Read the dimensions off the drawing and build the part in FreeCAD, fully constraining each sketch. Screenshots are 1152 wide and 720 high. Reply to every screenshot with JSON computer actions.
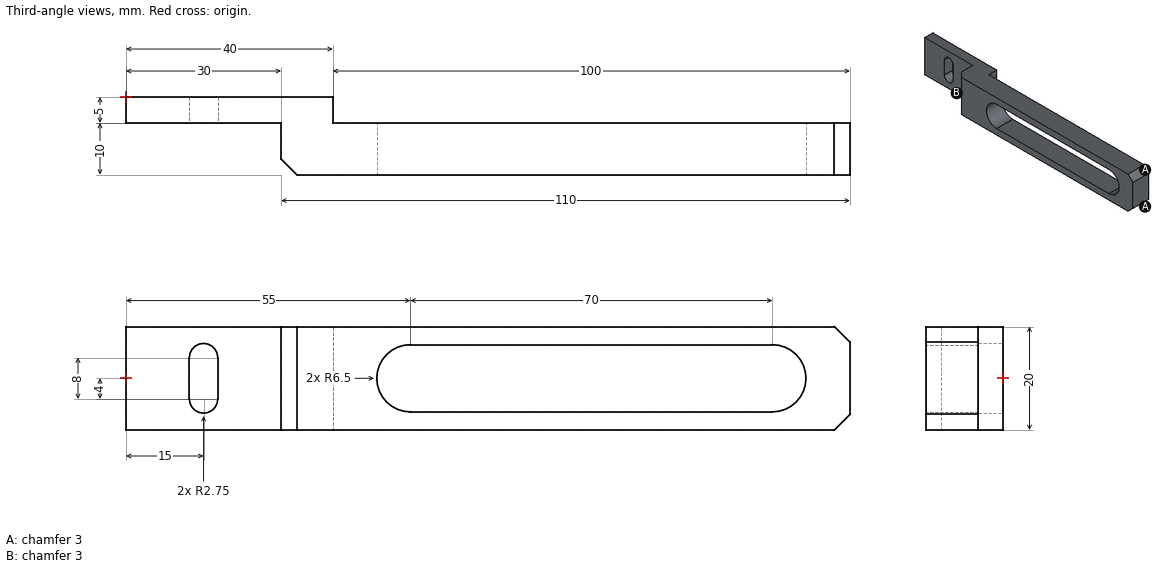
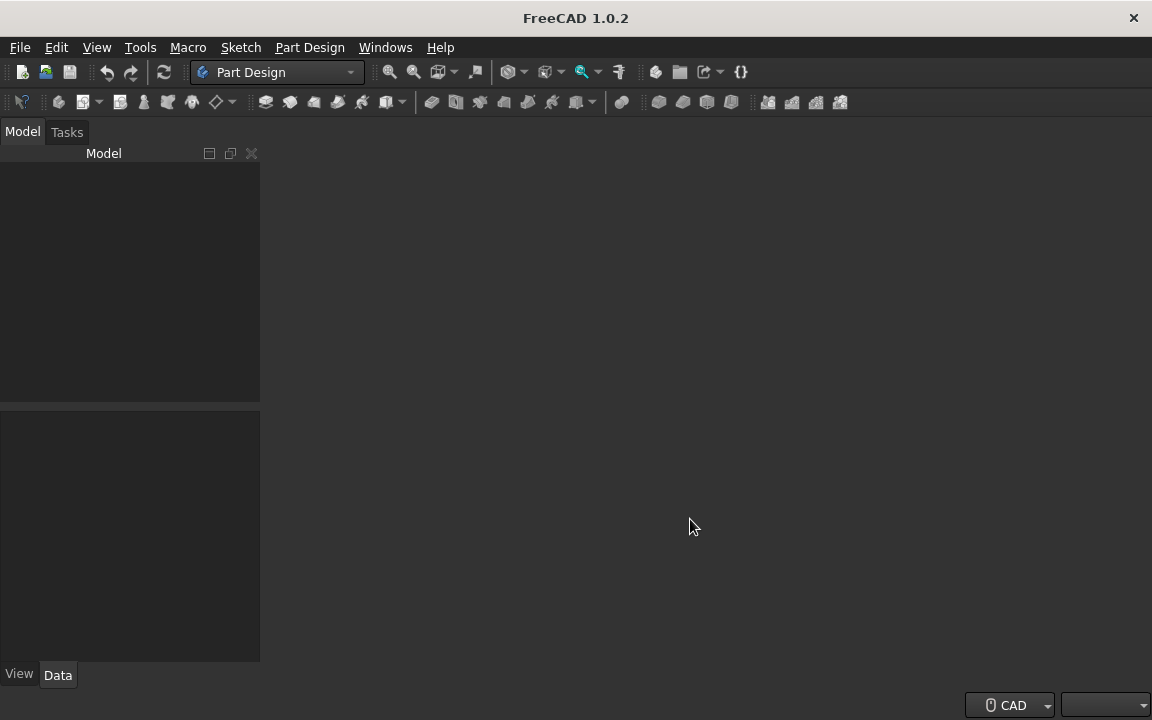
{"action": "left_click", "coordinate": [22, 72]}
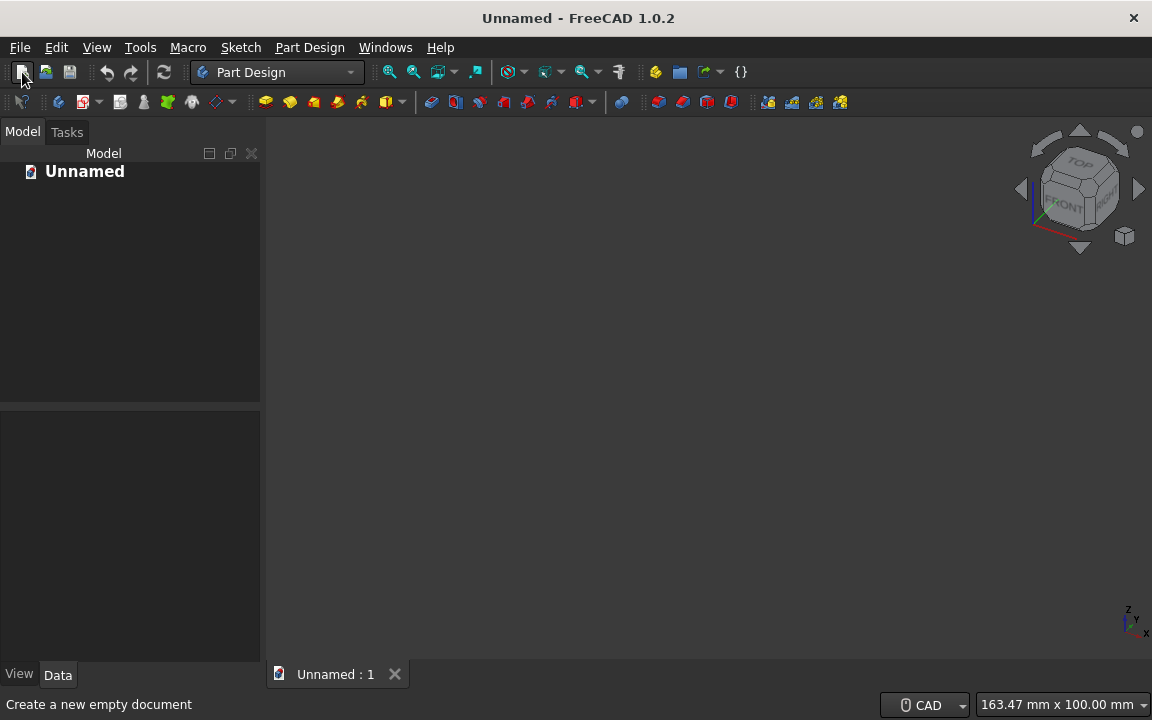
{"action": "left_click", "coordinate": [84, 102]}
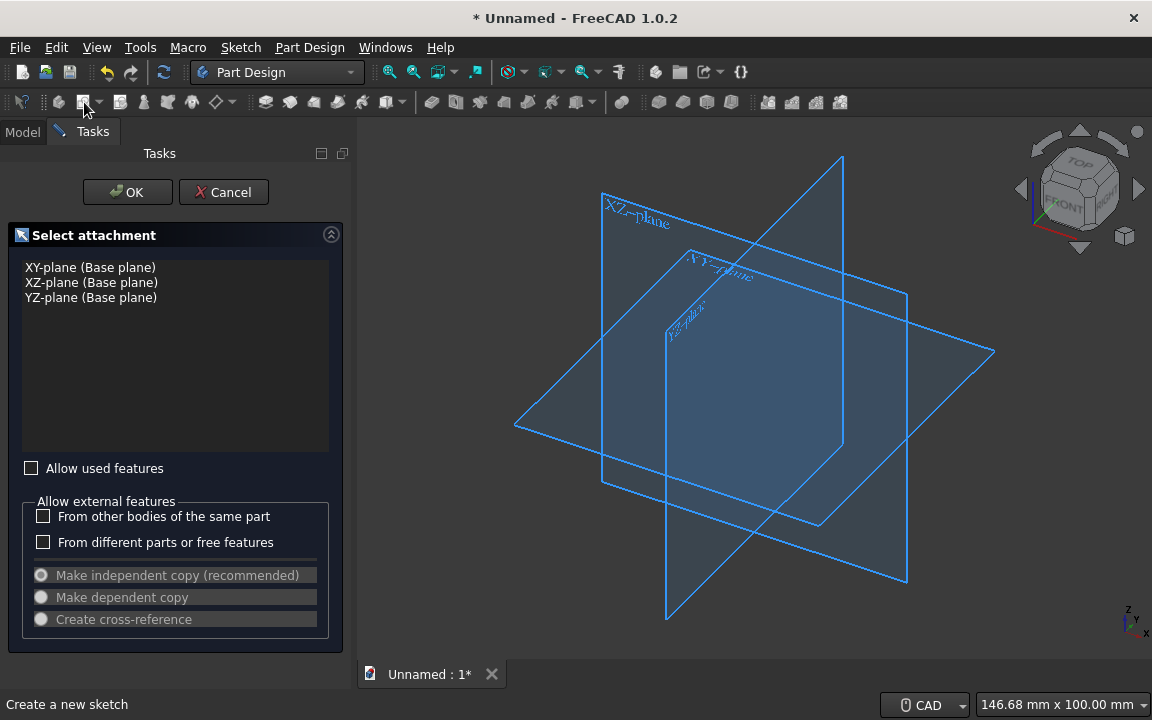
{"action": "left_click", "coordinate": [82, 268]}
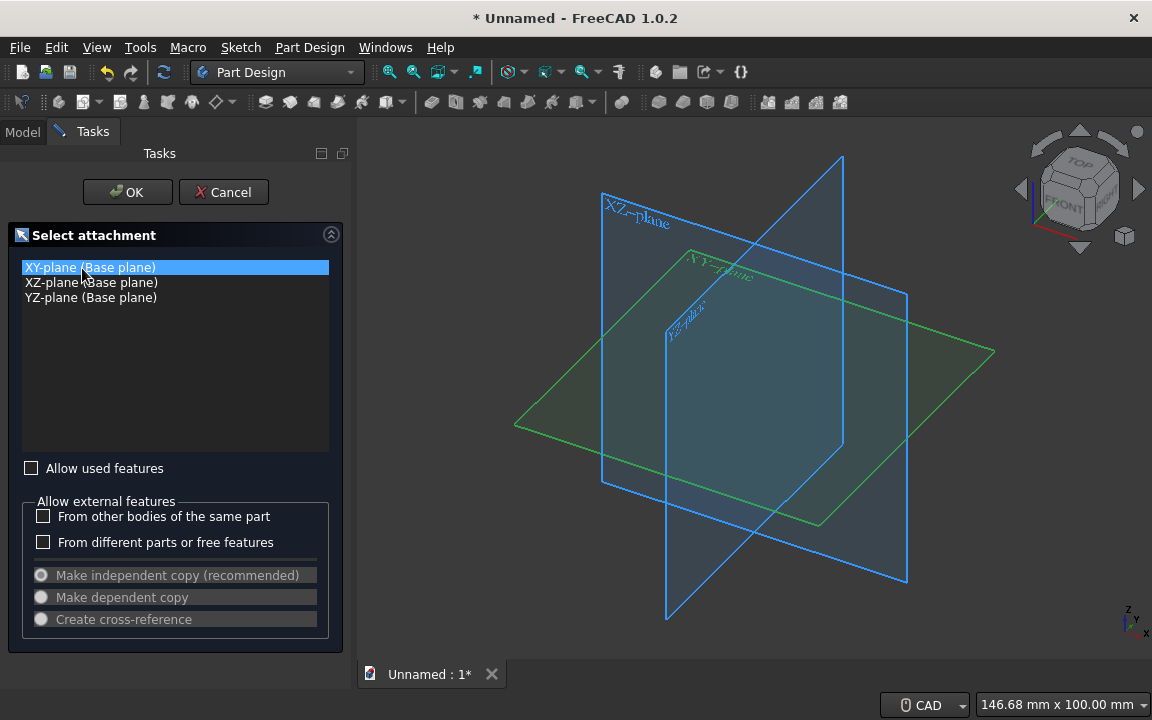
{"action": "left_click", "coordinate": [128, 192]}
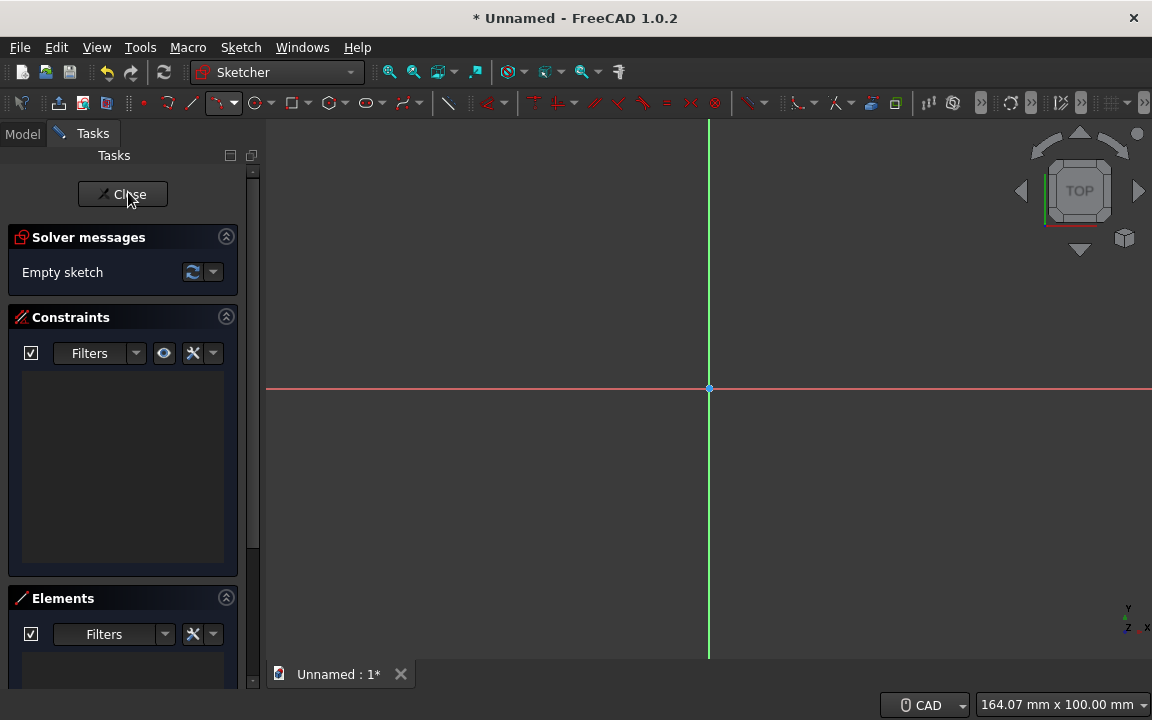
{"action": "scroll", "coordinate": [294, 340], "scroll_direction": "down", "scroll_amount": 3}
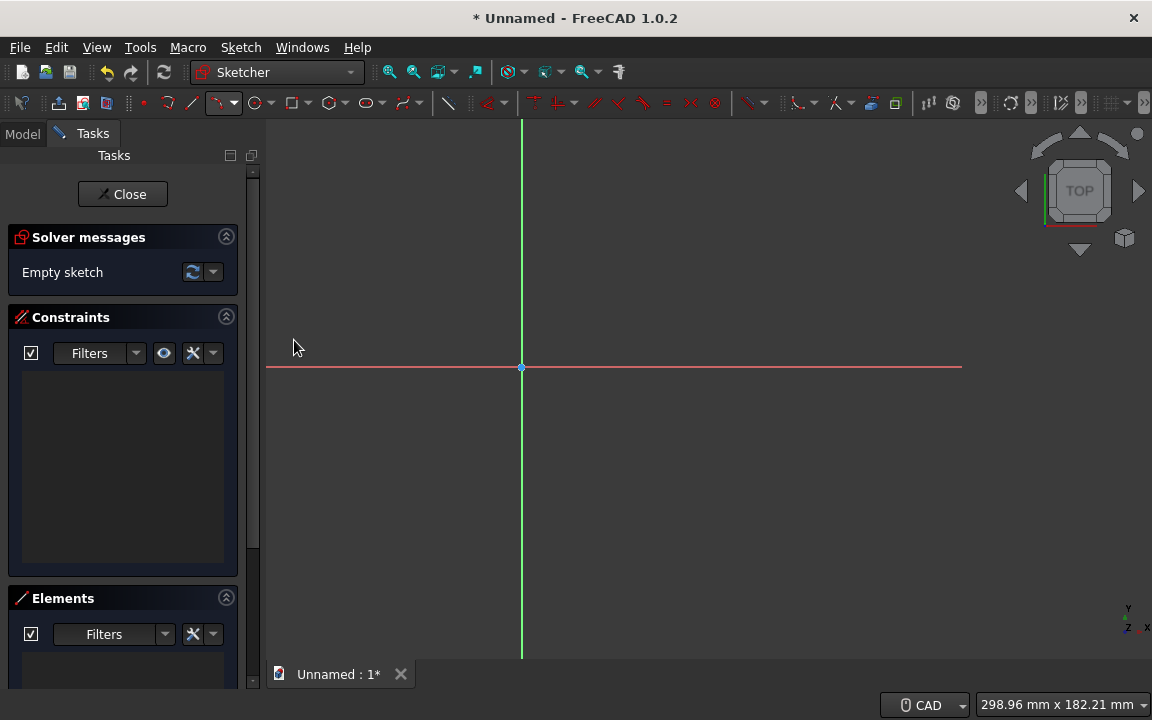
{"action": "key", "text": "g m"}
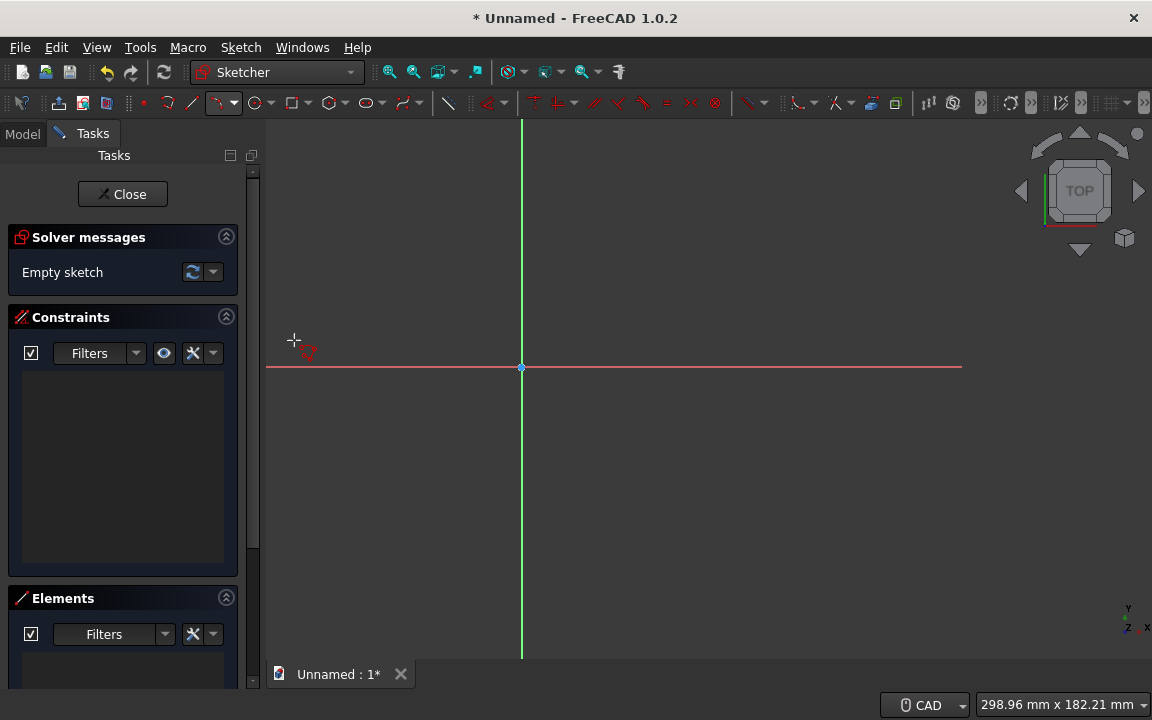
{"action": "left_click", "coordinate": [522, 367]}
{"action": "left_click", "coordinate": [531, 382]}
{"action": "left_click", "coordinate": [611, 382]}
{"action": "left_click", "coordinate": [611, 412]}
{"action": "left_click", "coordinate": [937, 412]}
{"action": "left_click", "coordinate": [937, 376]}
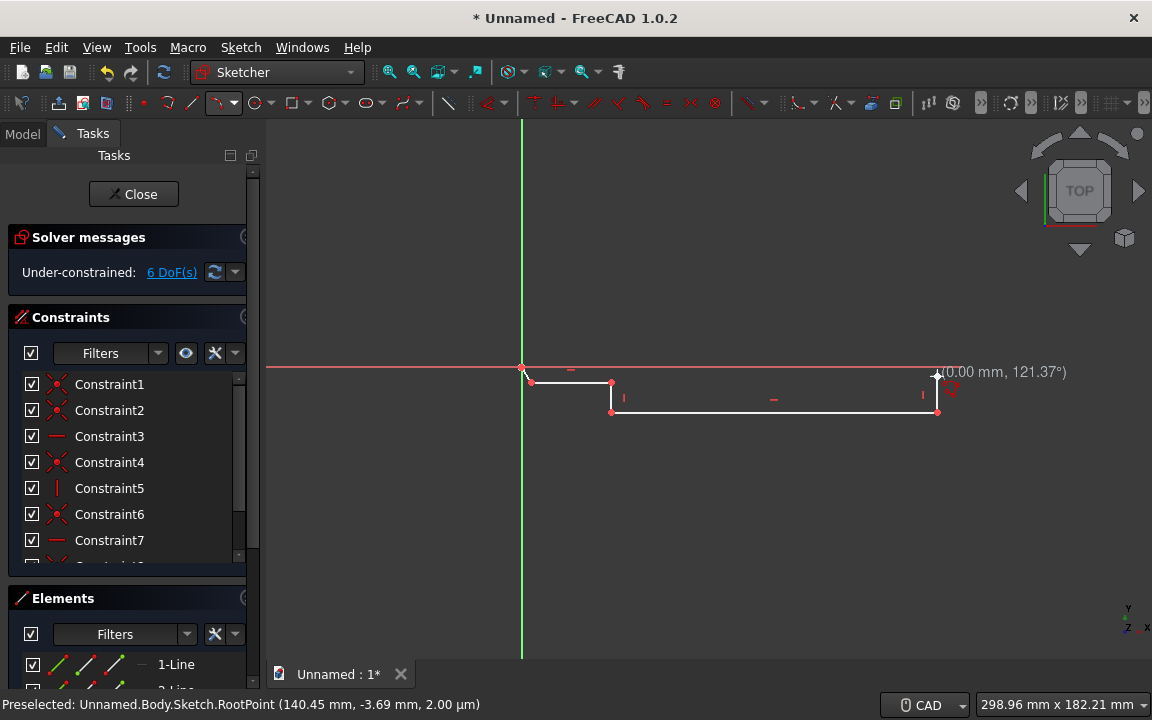
{"action": "scroll", "coordinate": [522, 367], "scroll_direction": "up", "scroll_amount": 4}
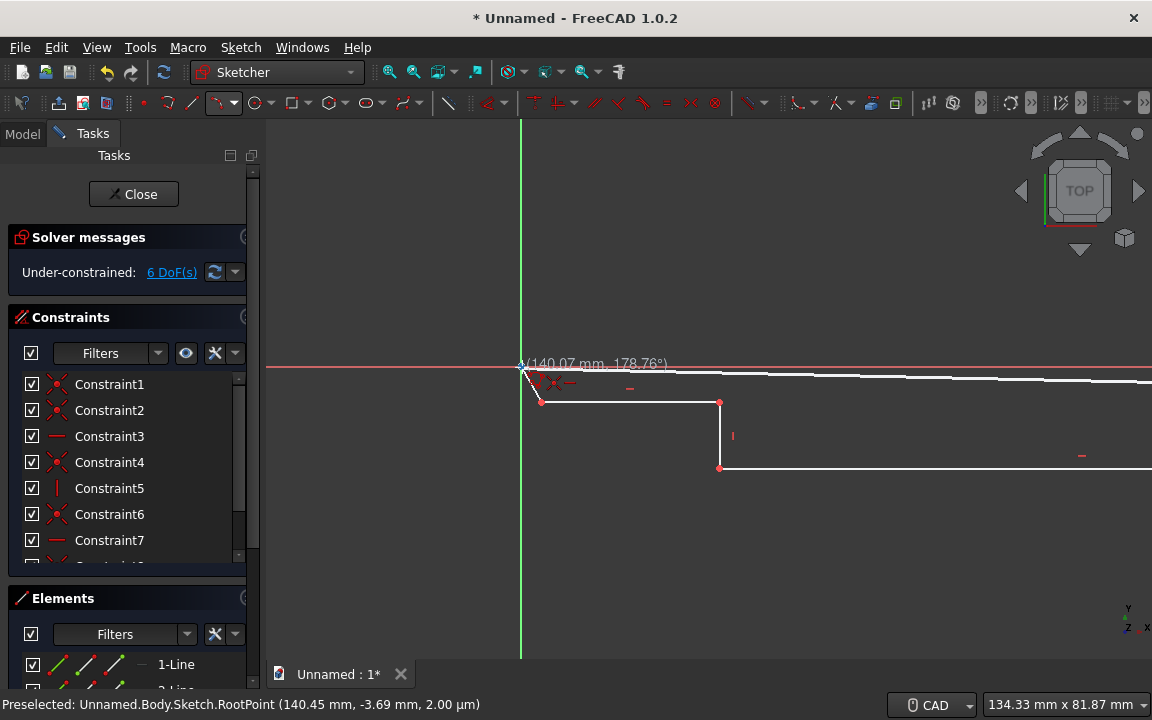
{"action": "left_click", "coordinate": [521, 367]}
{"action": "key", "text": "Escape"}
{"action": "key", "text": "Escape"}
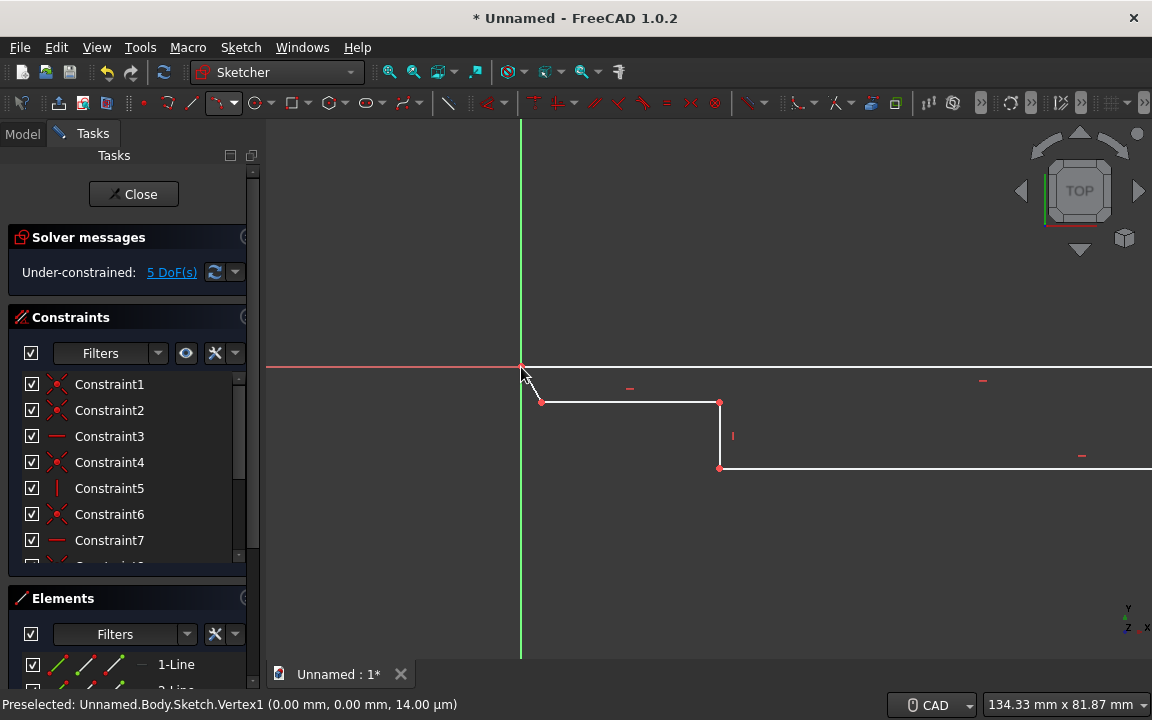
{"action": "left_click", "coordinate": [536, 391]}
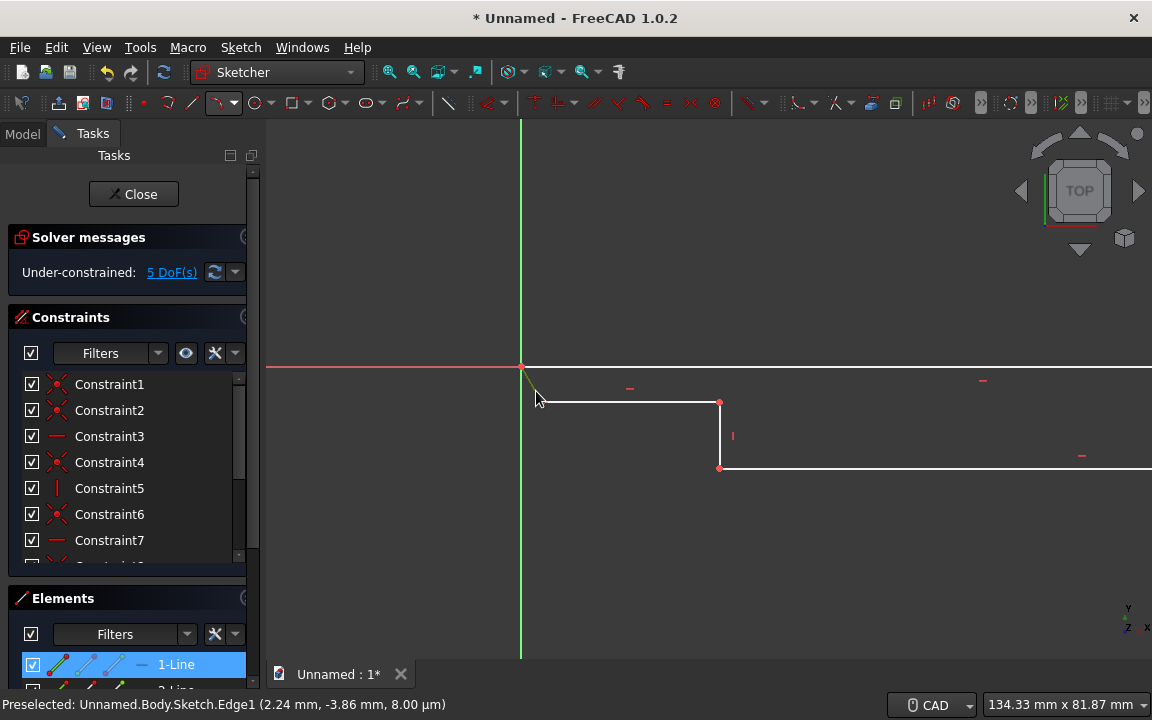
{"action": "key", "text": "v"}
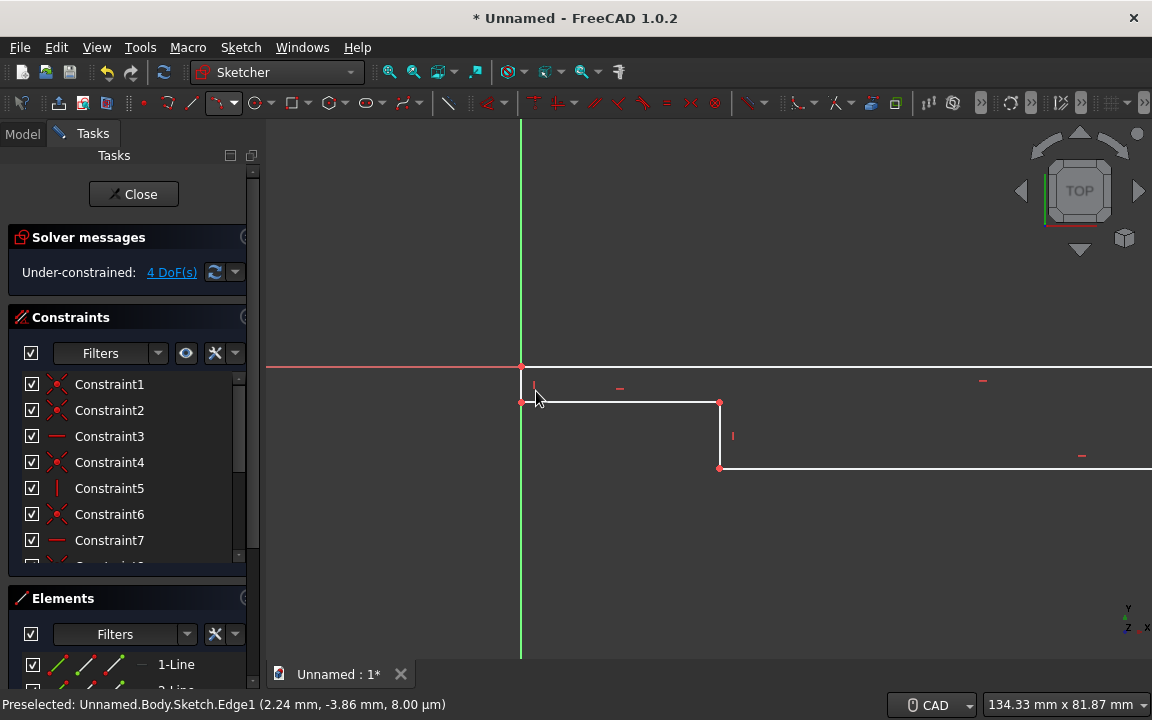
{"action": "scroll", "coordinate": [521, 377], "scroll_direction": "up", "scroll_amount": 2}